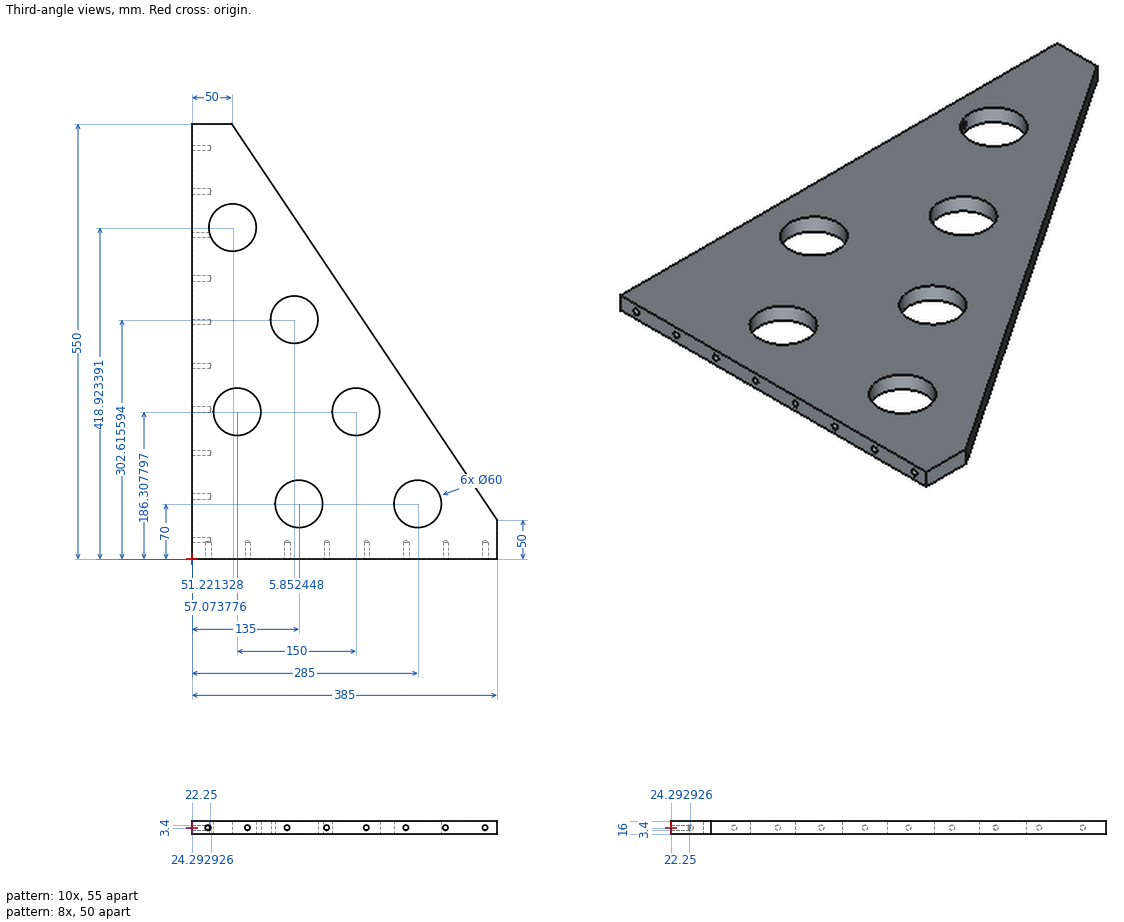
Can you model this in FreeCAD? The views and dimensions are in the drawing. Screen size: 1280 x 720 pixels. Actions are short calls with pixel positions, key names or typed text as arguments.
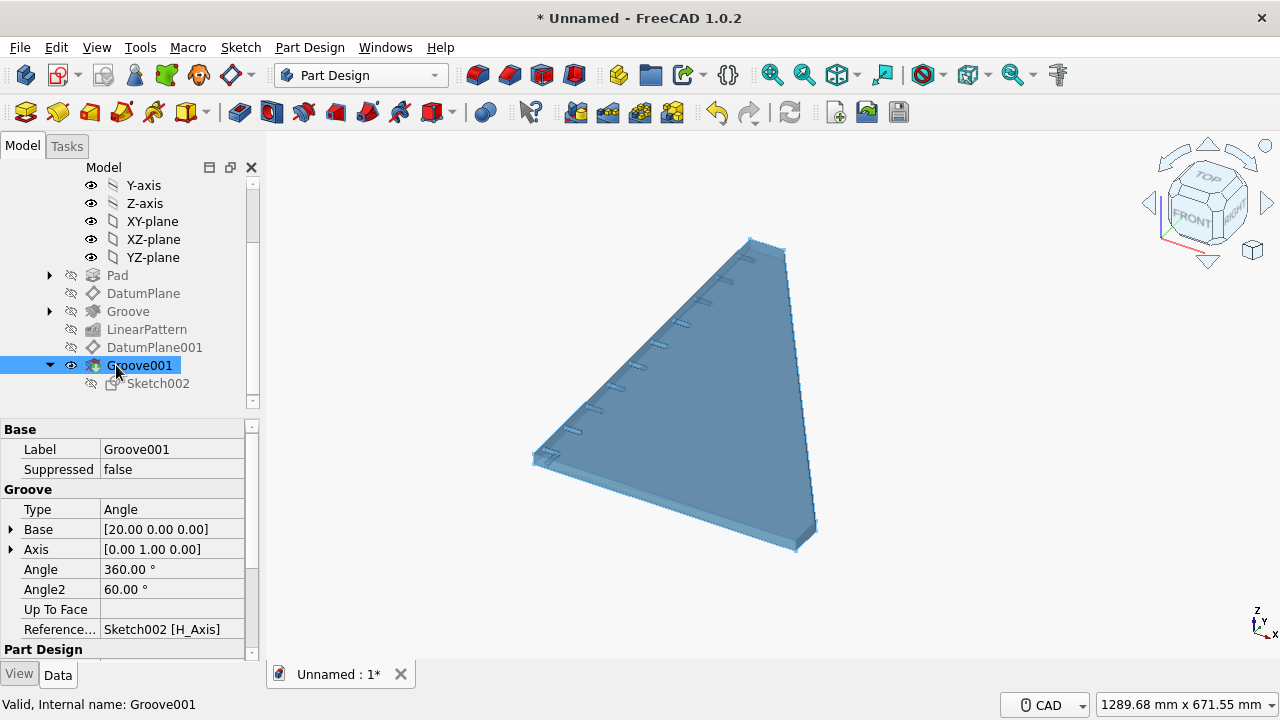
click(608, 112)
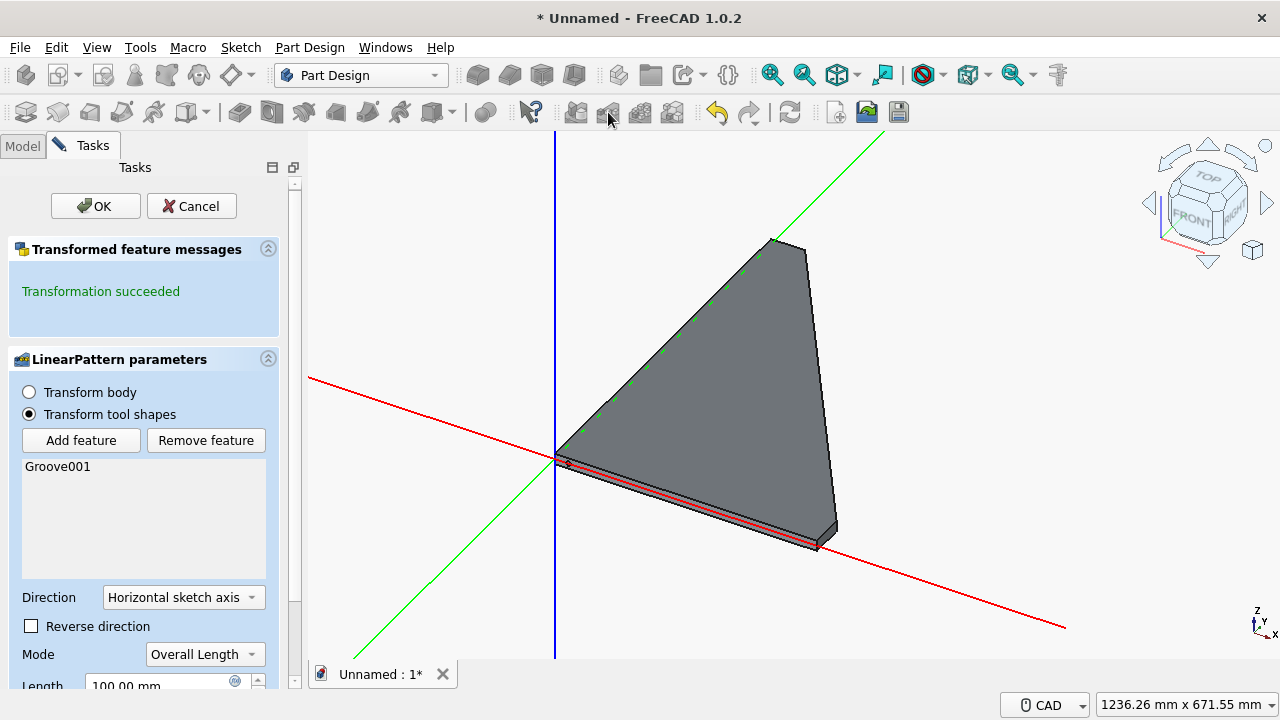
click(184, 598)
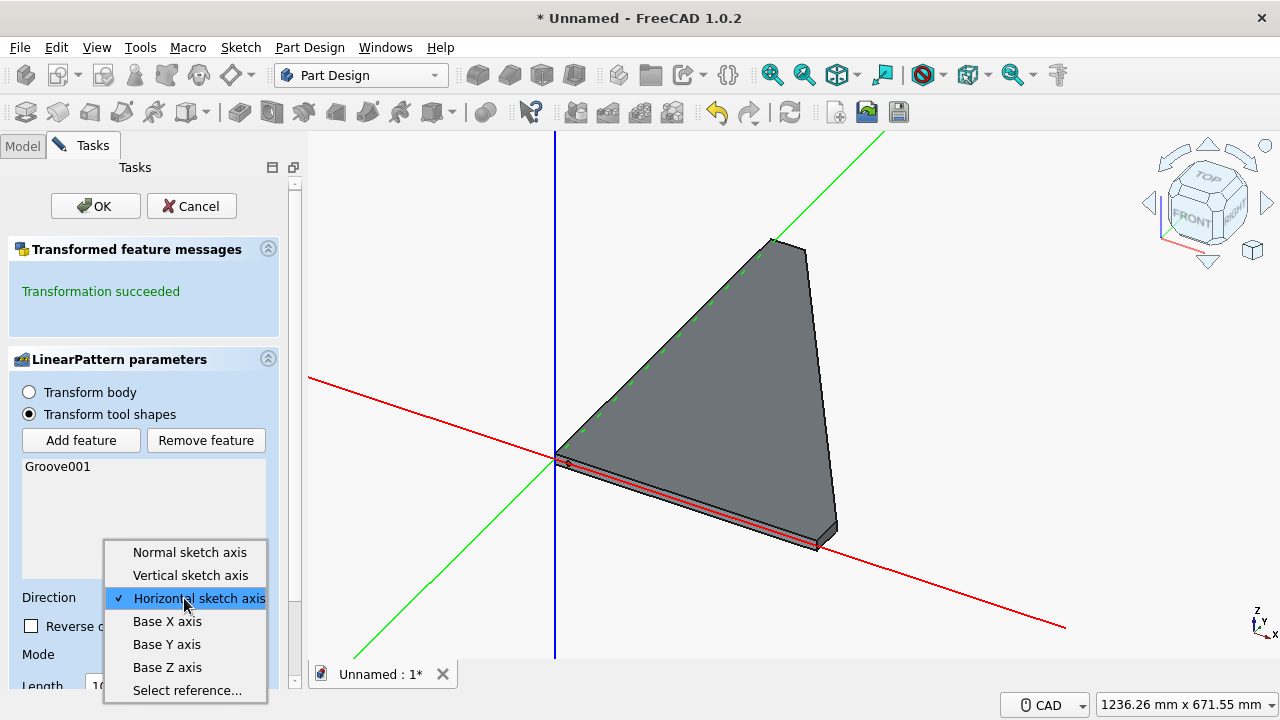
click(184, 622)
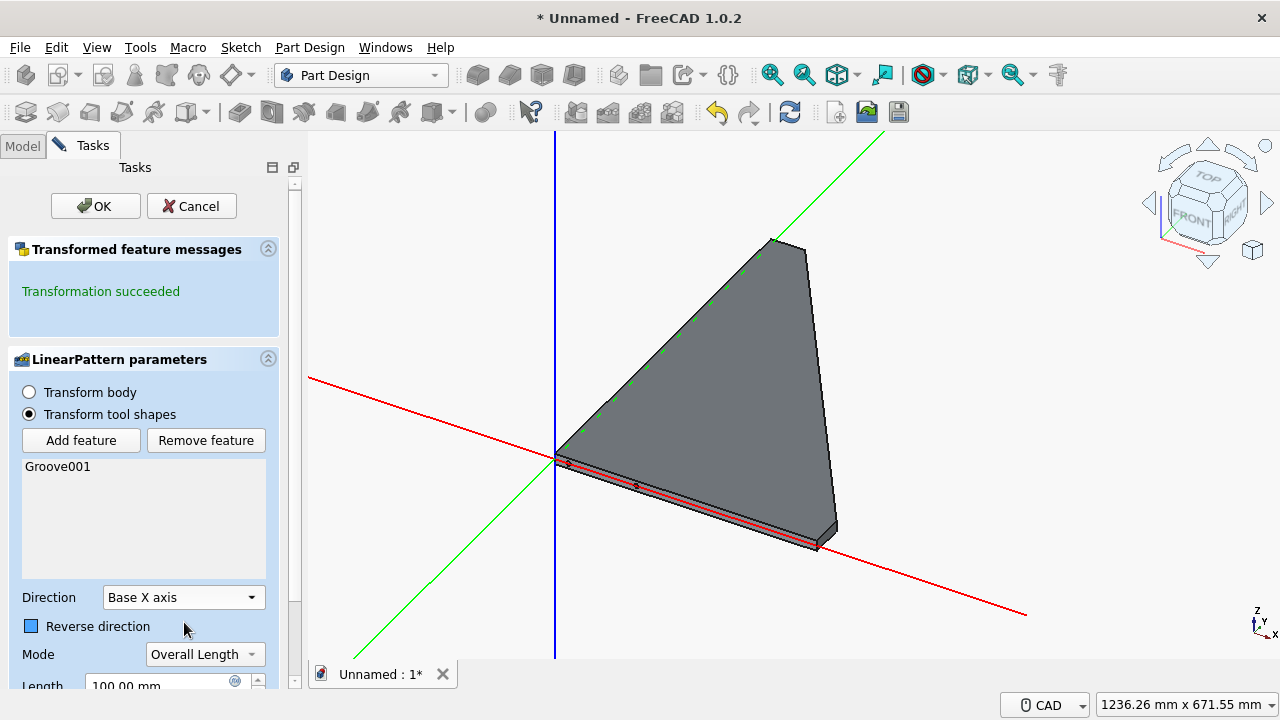
click(206, 654)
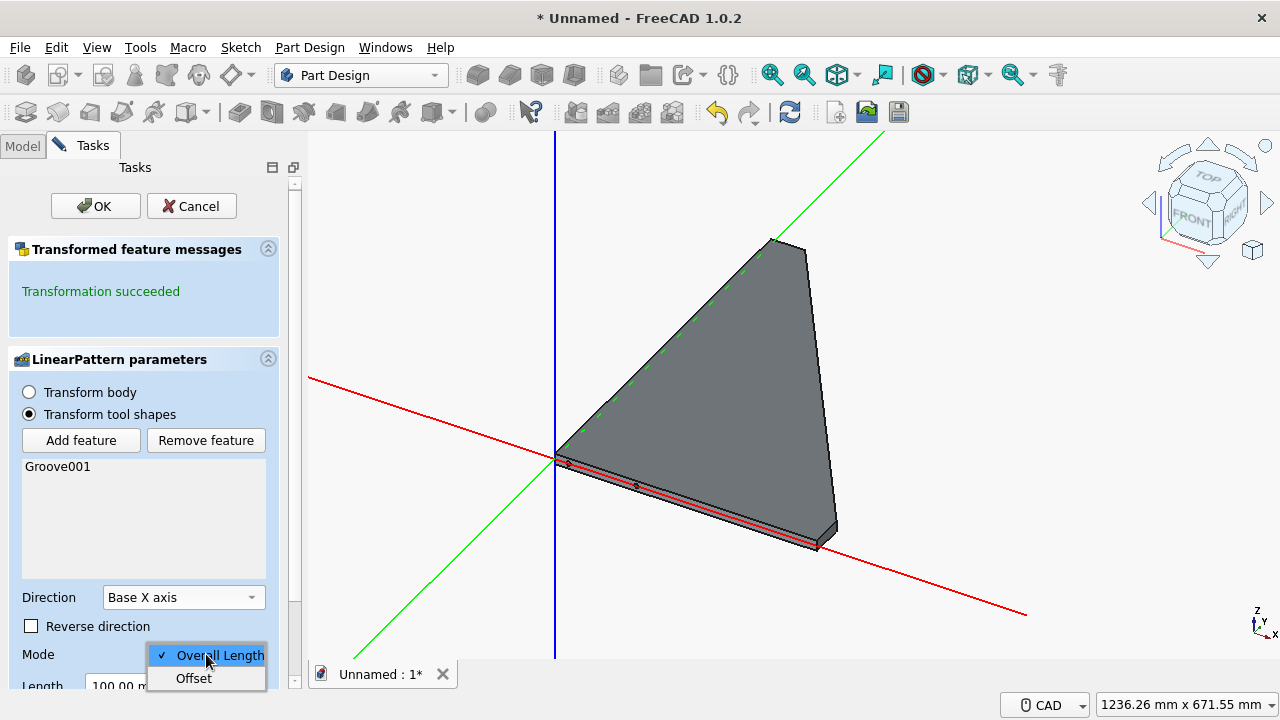
click(206, 678)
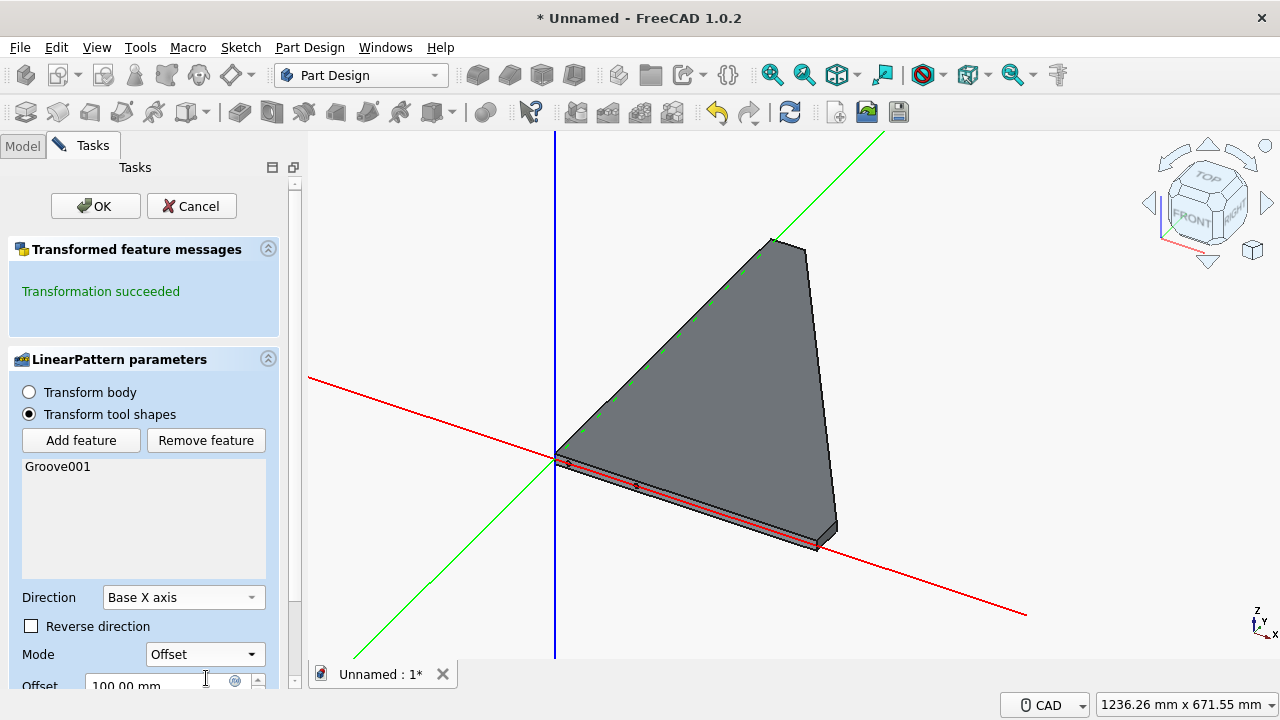
scroll(295, 432, down, 2)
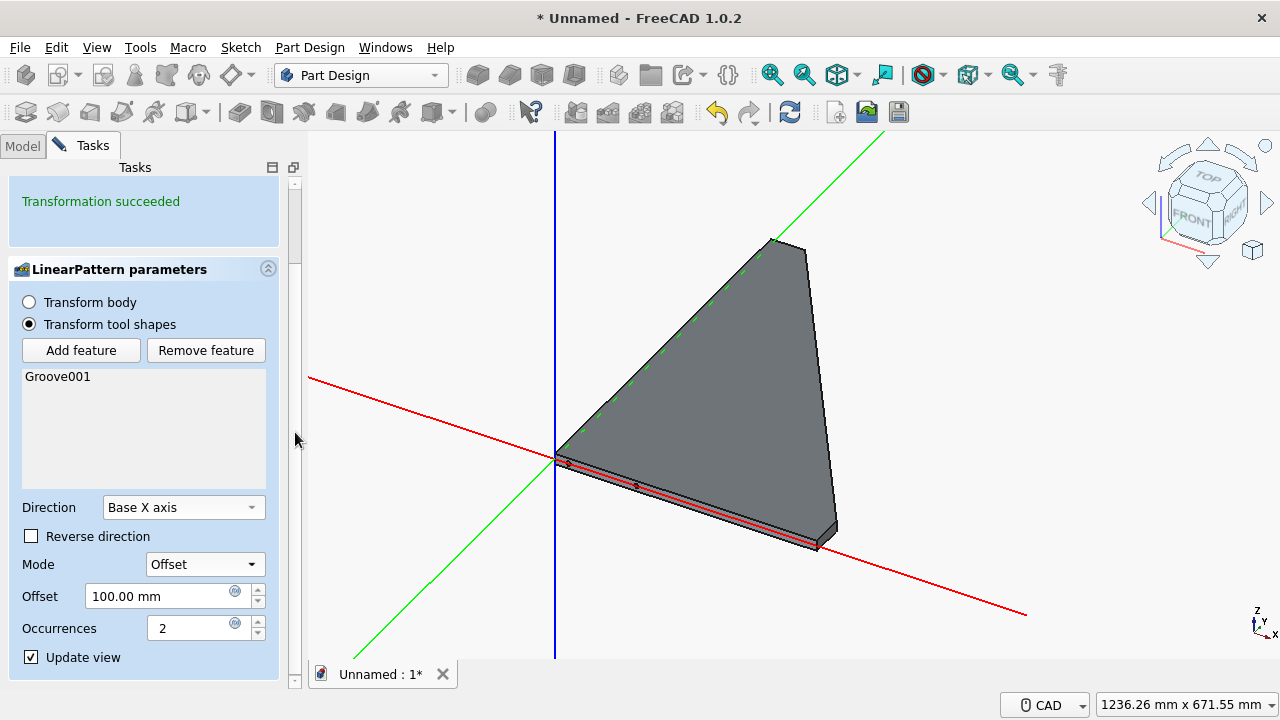
triple_click(168, 596)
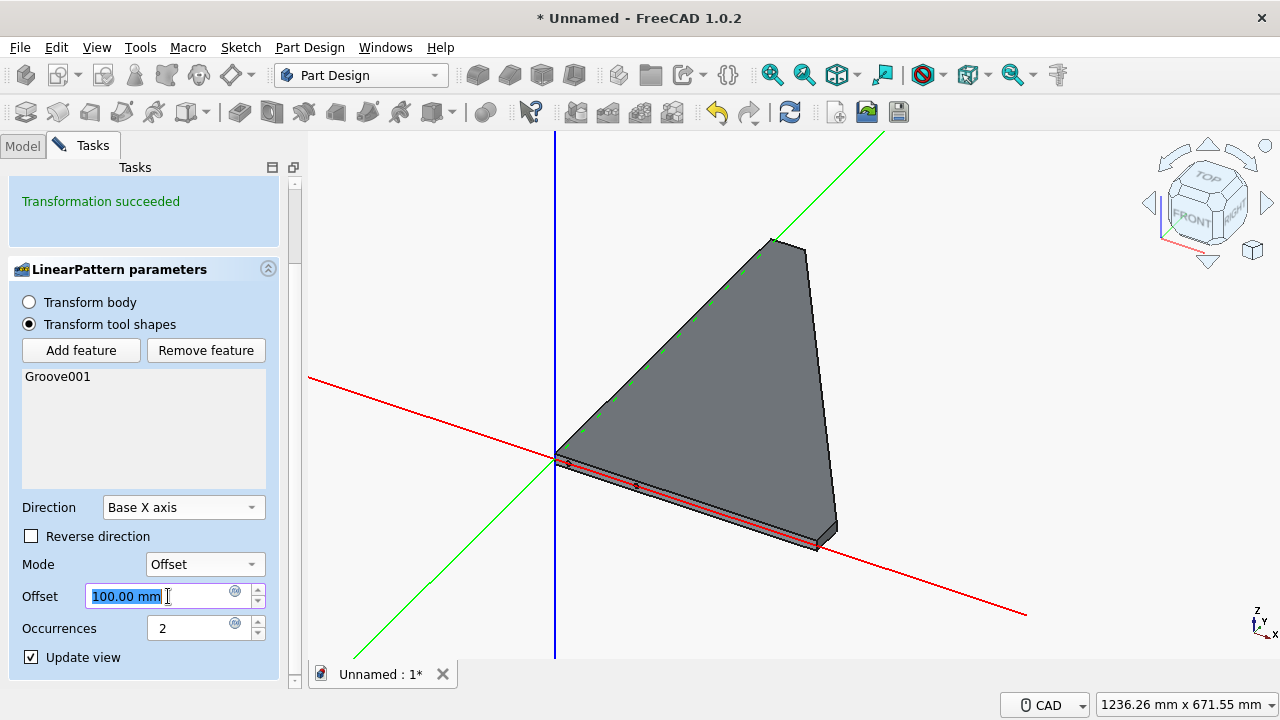
text(50)
key(Tab)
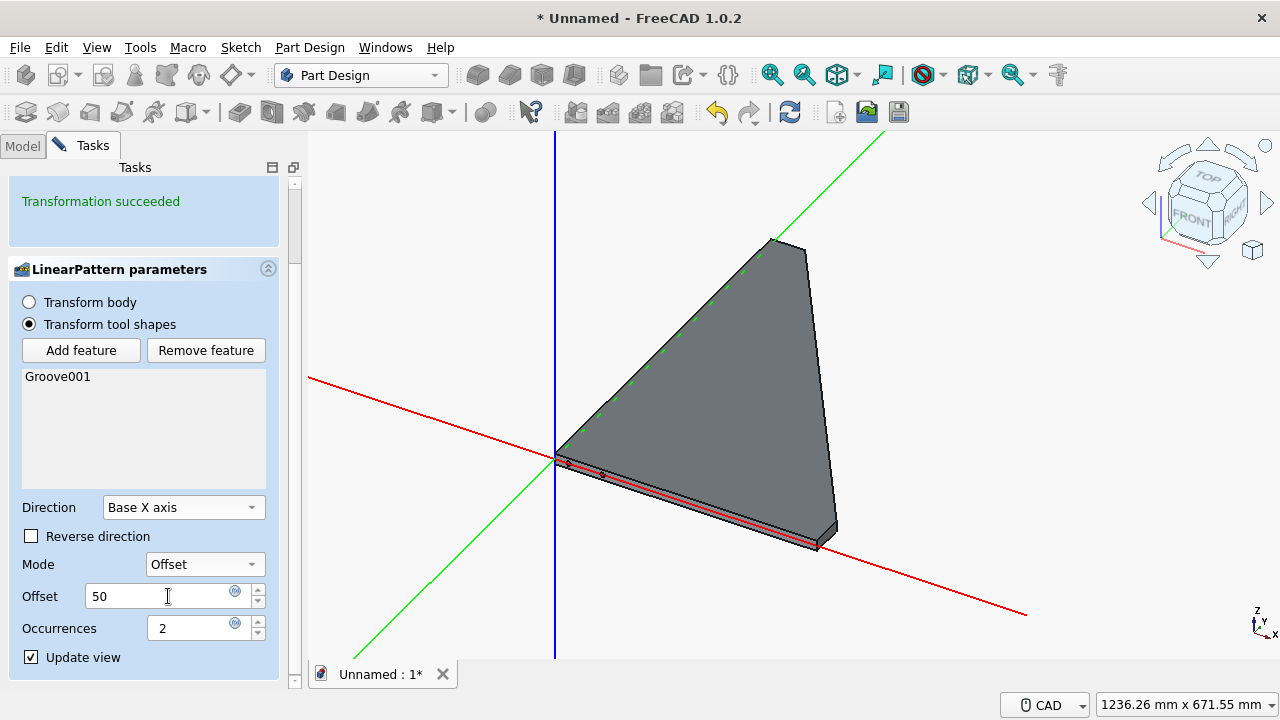
triple_click(198, 628)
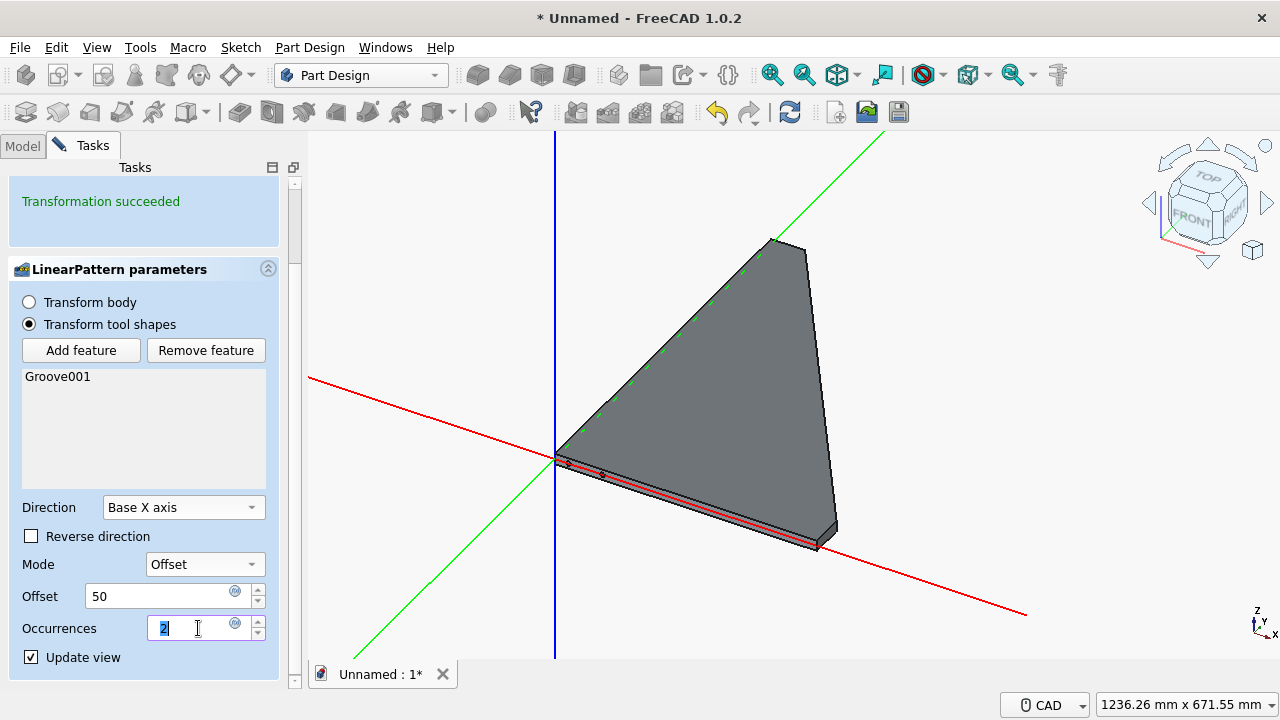
text(8)
key(Tab)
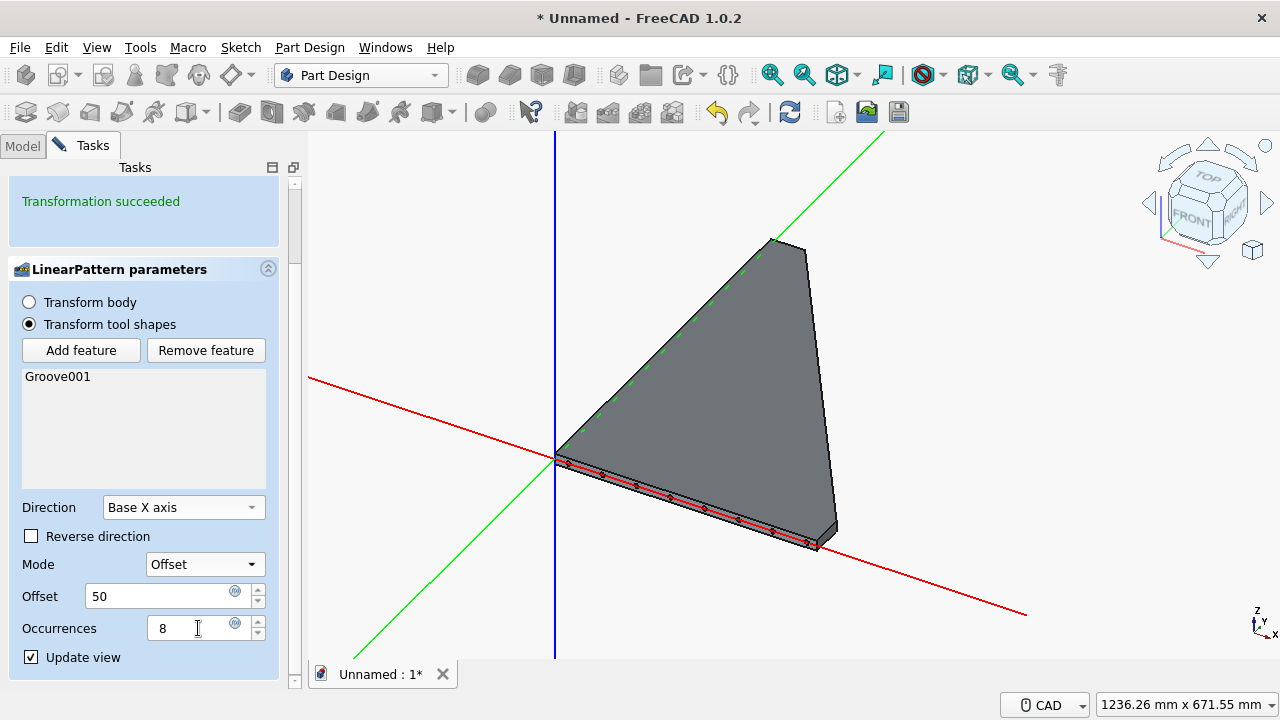
scroll(295, 432, up, 3)